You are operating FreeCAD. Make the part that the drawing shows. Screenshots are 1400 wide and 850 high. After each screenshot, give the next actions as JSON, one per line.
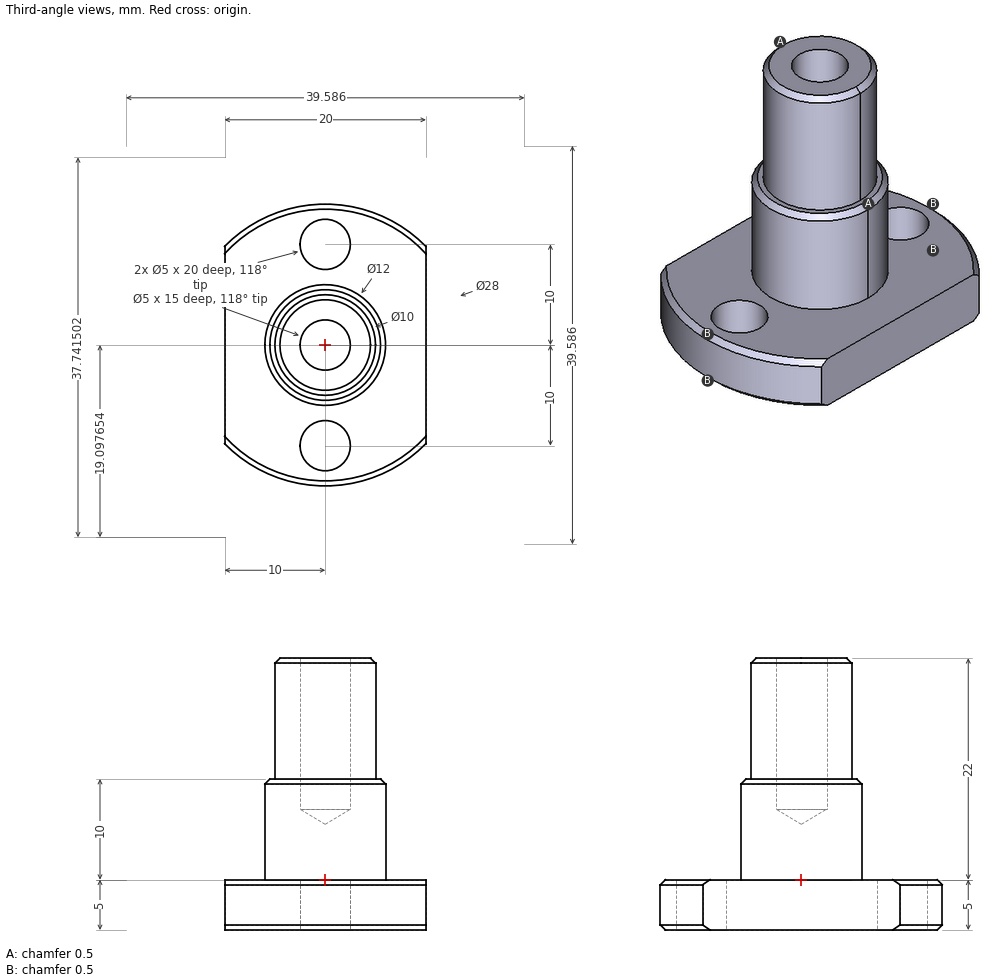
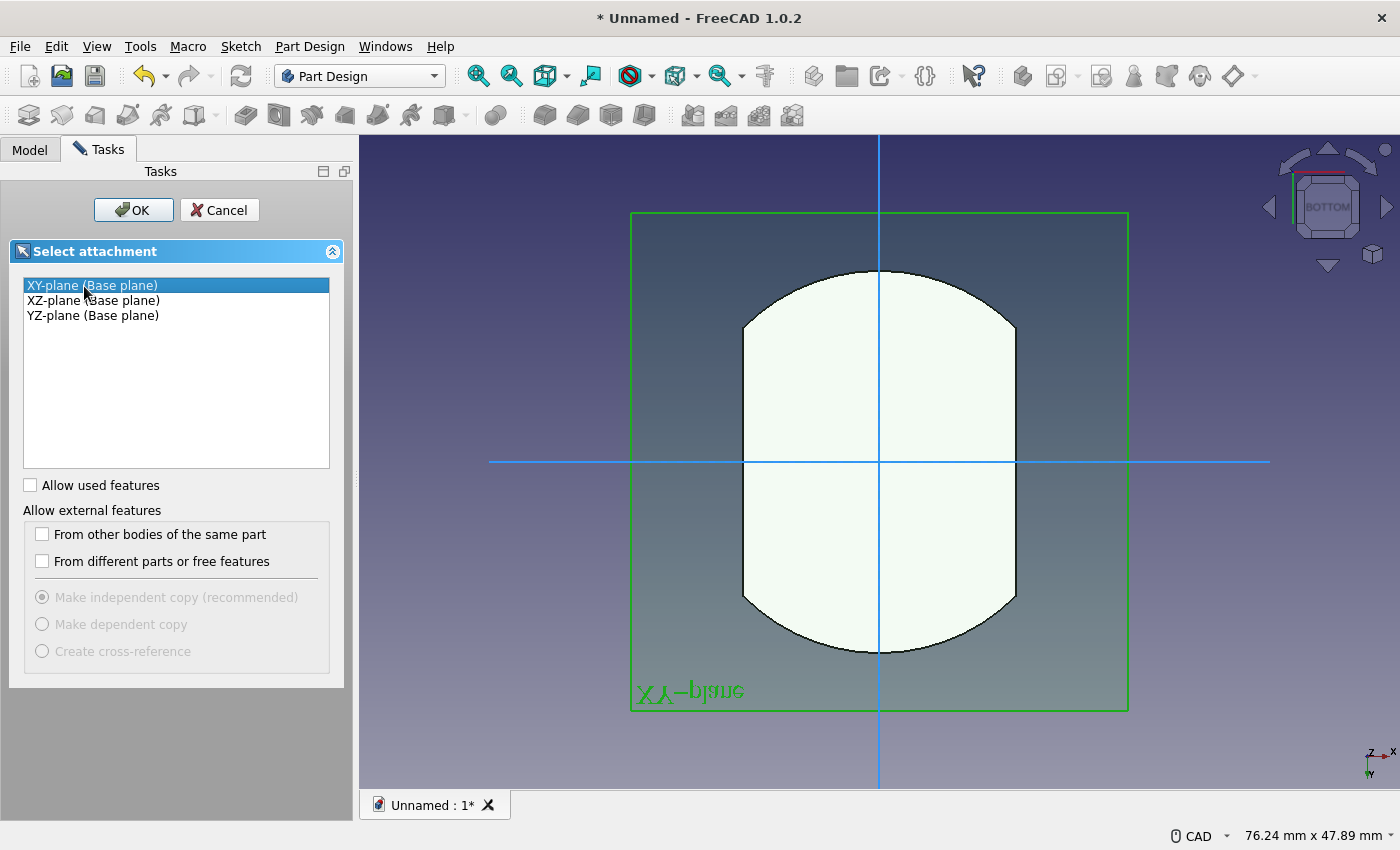
{"action": "left_click", "coordinate": [134, 210]}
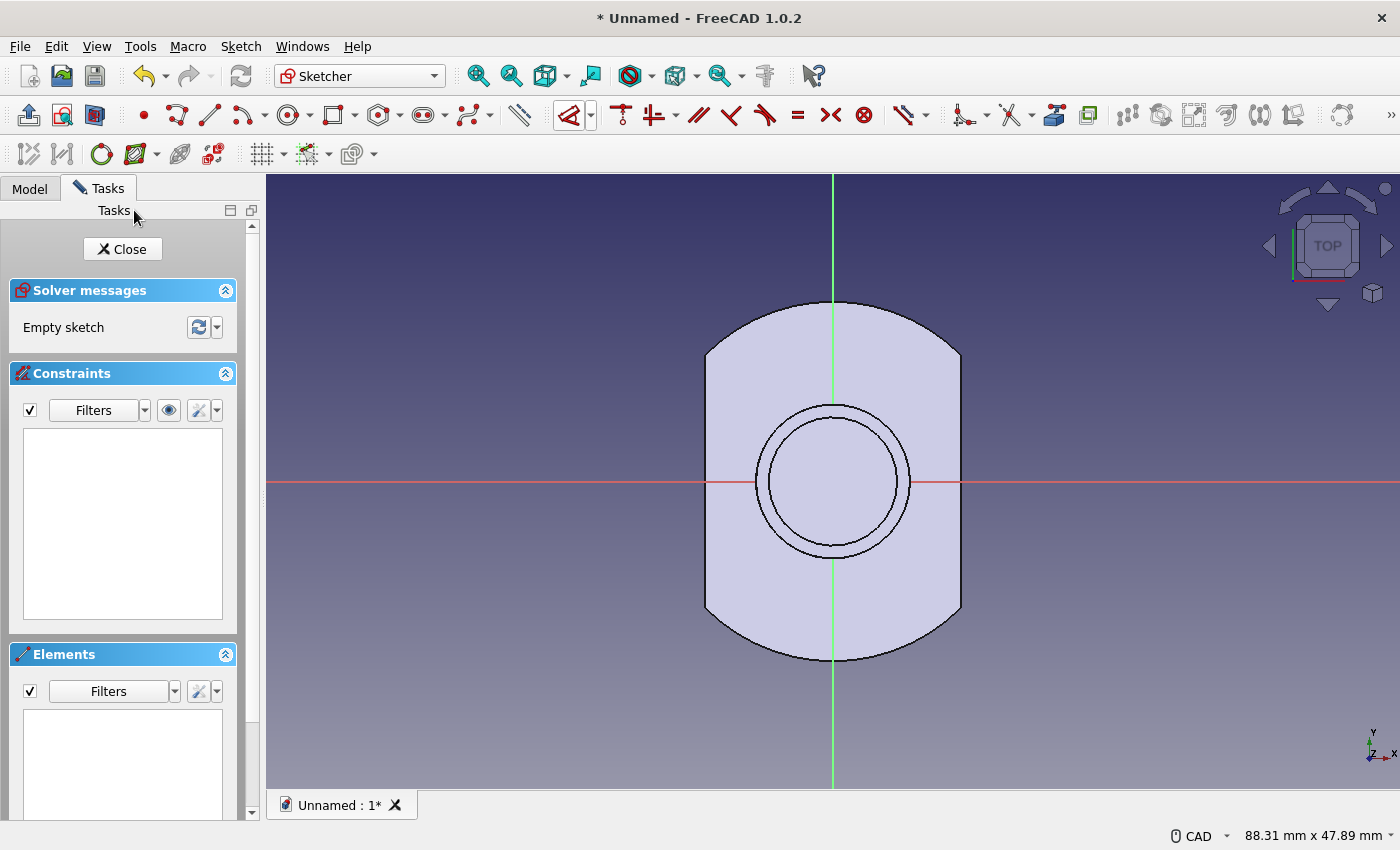
{"action": "key", "text": "q s"}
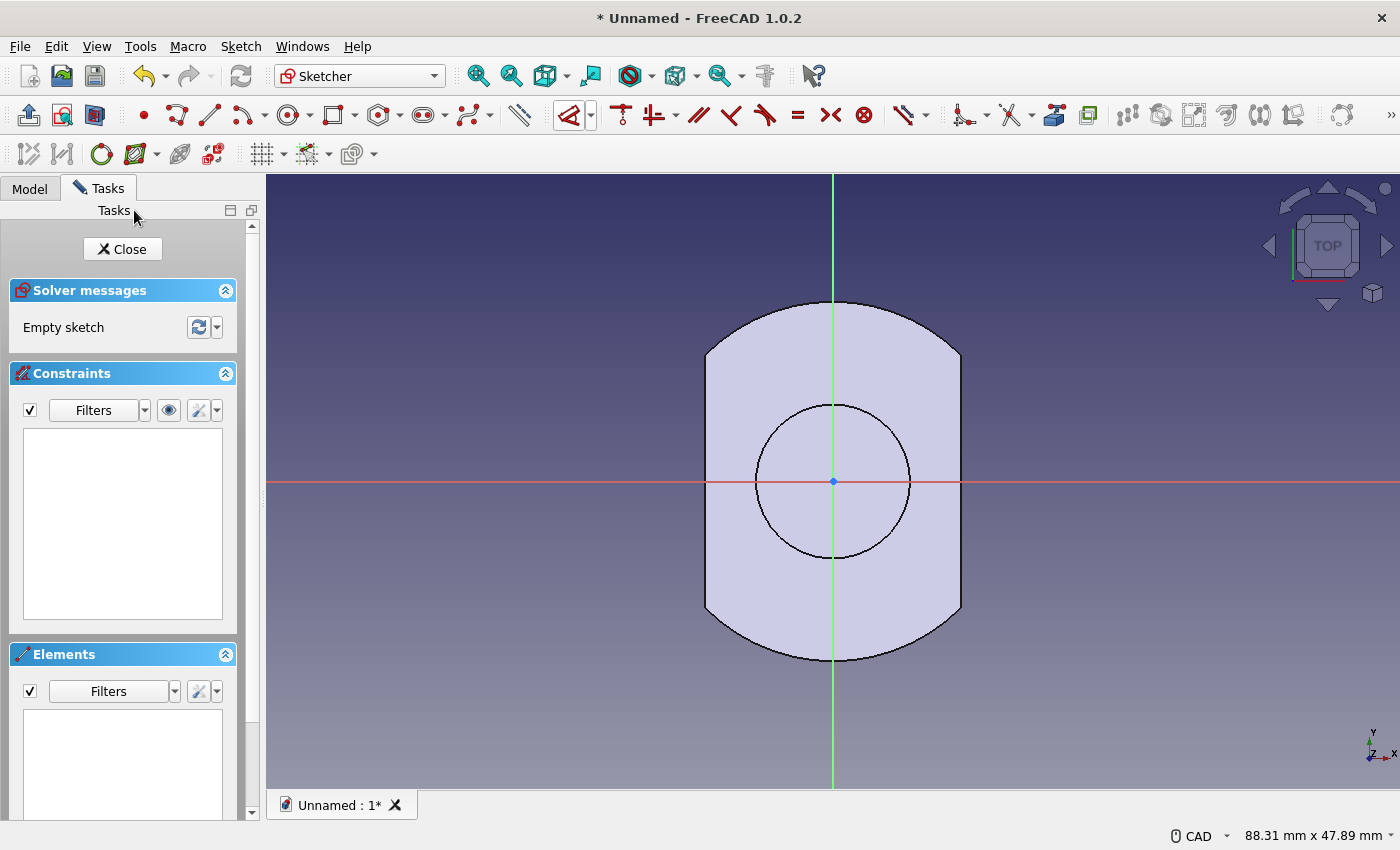
{"action": "left_click", "coordinate": [288, 116]}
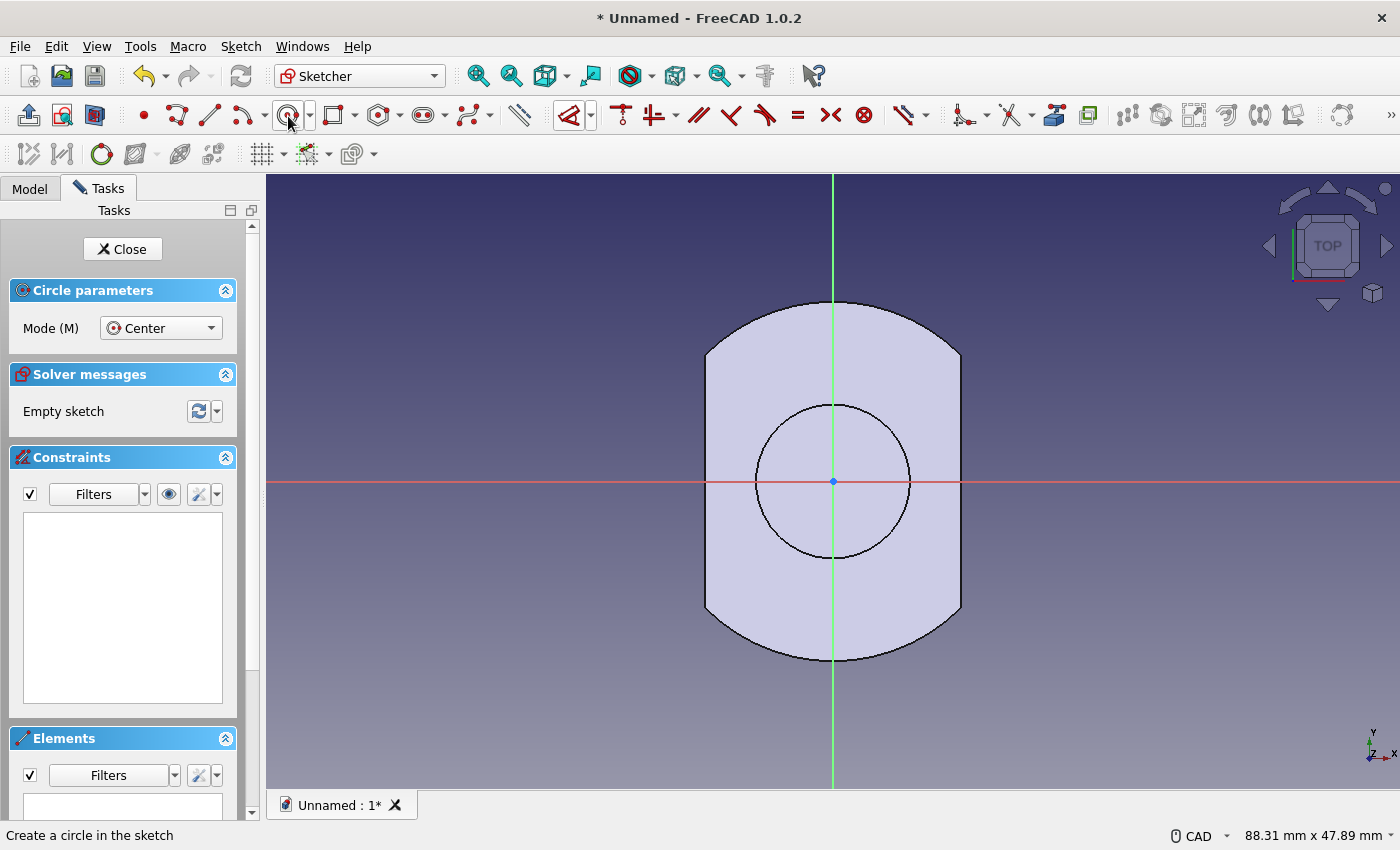
{"action": "left_click", "coordinate": [833, 353]}
{"action": "mouse_move", "coordinate": [856, 330]}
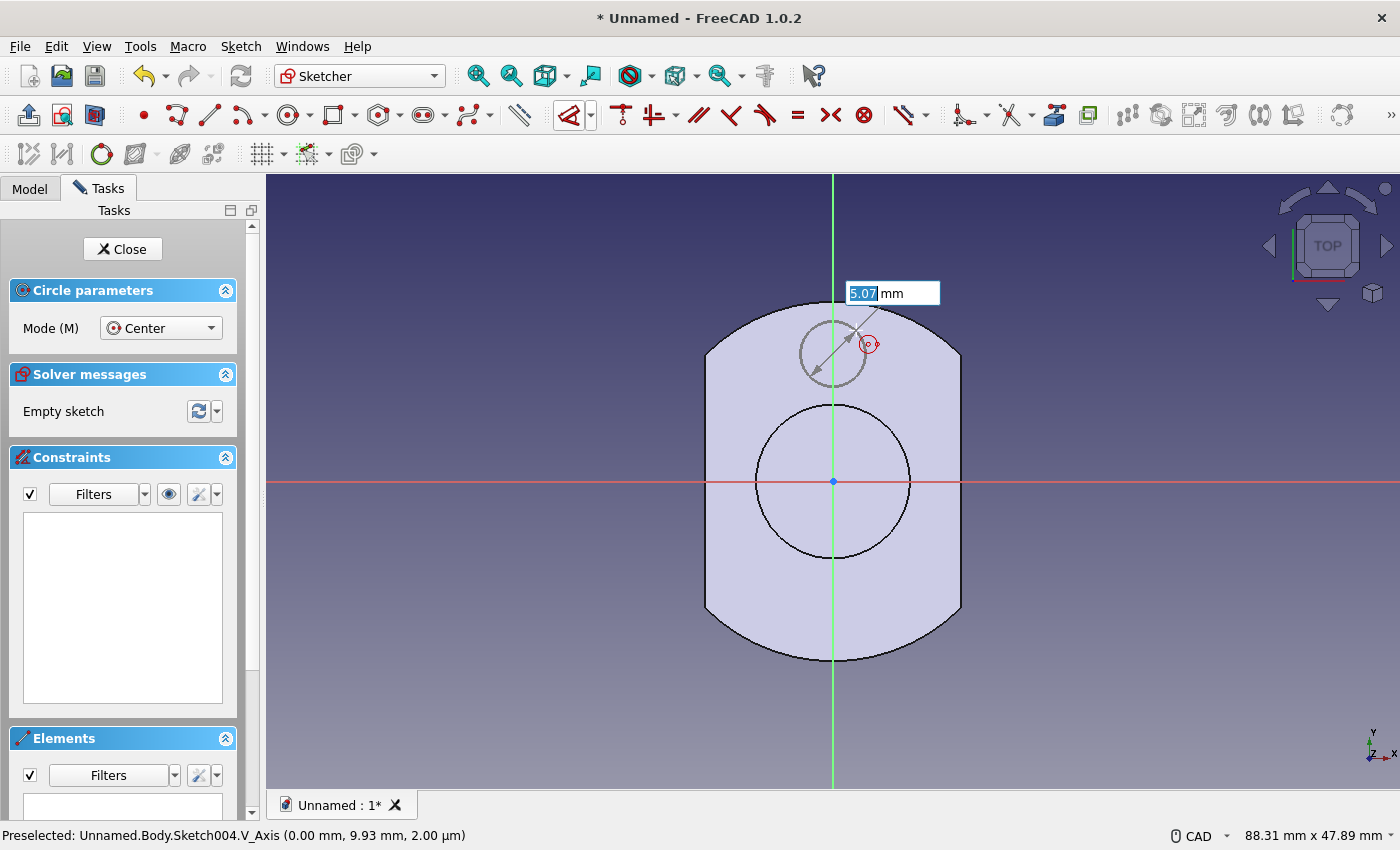
{"action": "type", "text": "5"}
{"action": "key", "text": "Return"}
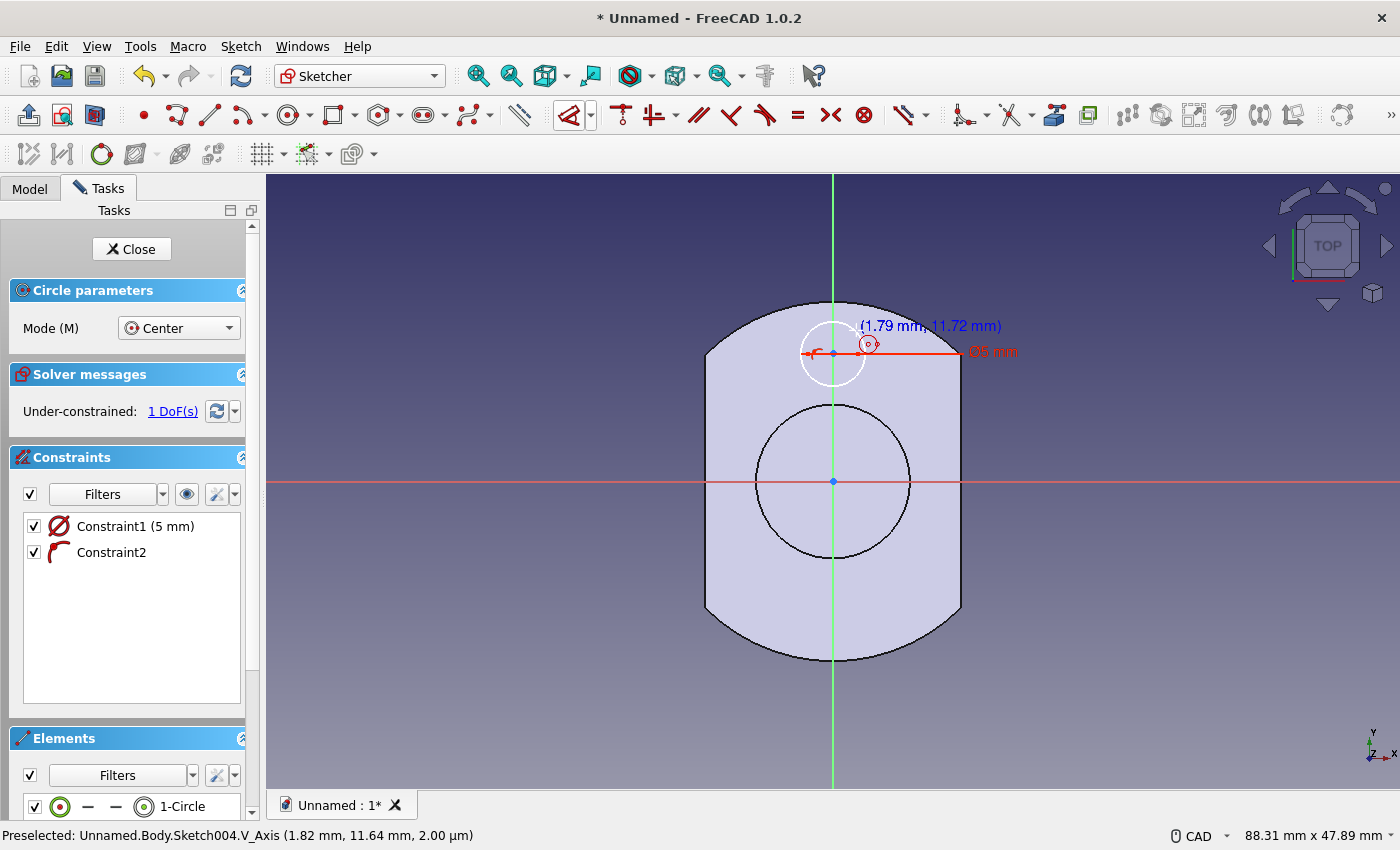
{"action": "left_click", "coordinate": [833, 610]}
{"action": "mouse_move", "coordinate": [856, 587]}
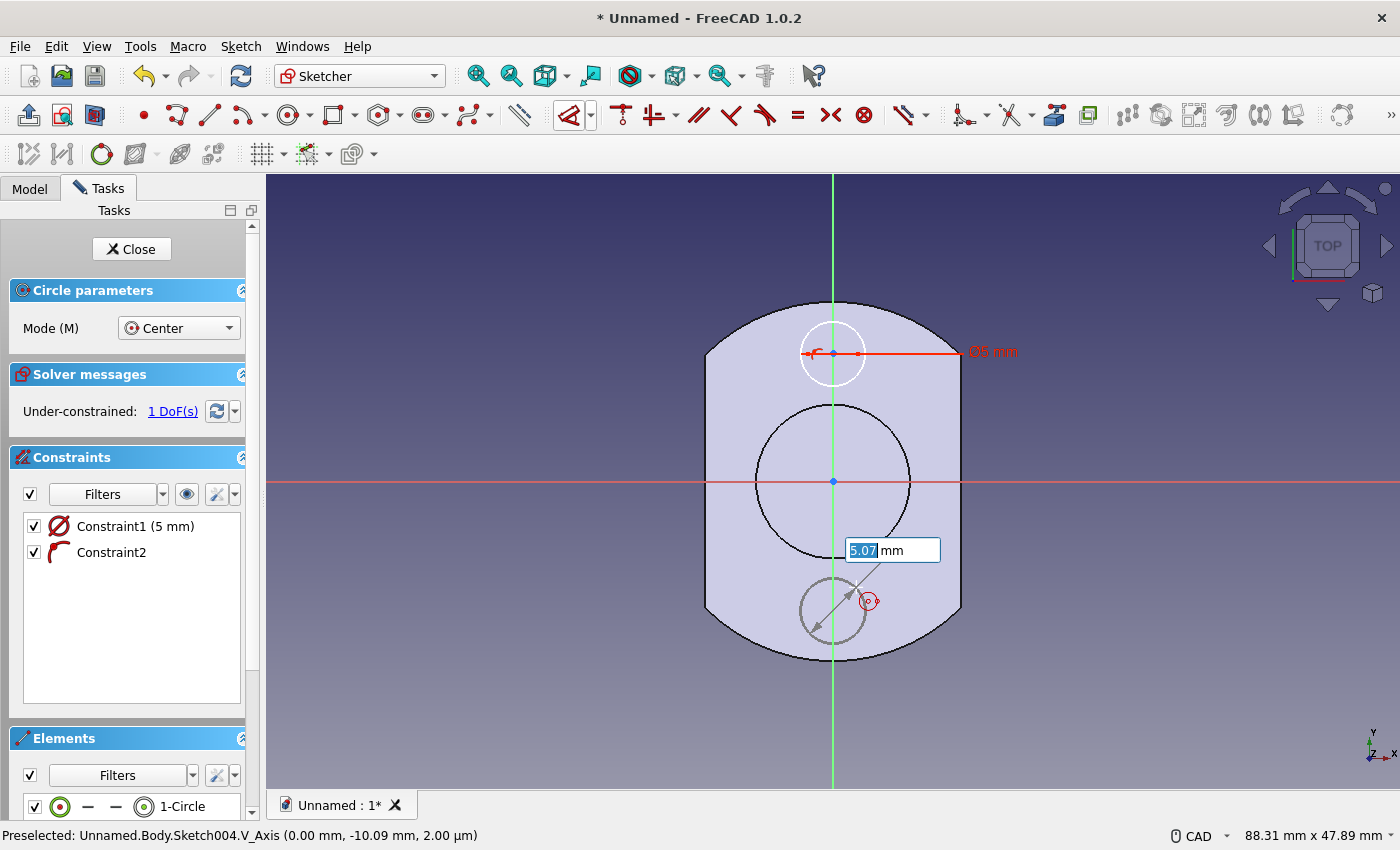
{"action": "type", "text": "5"}
{"action": "key", "text": "Return"}
{"action": "key", "text": "Escape"}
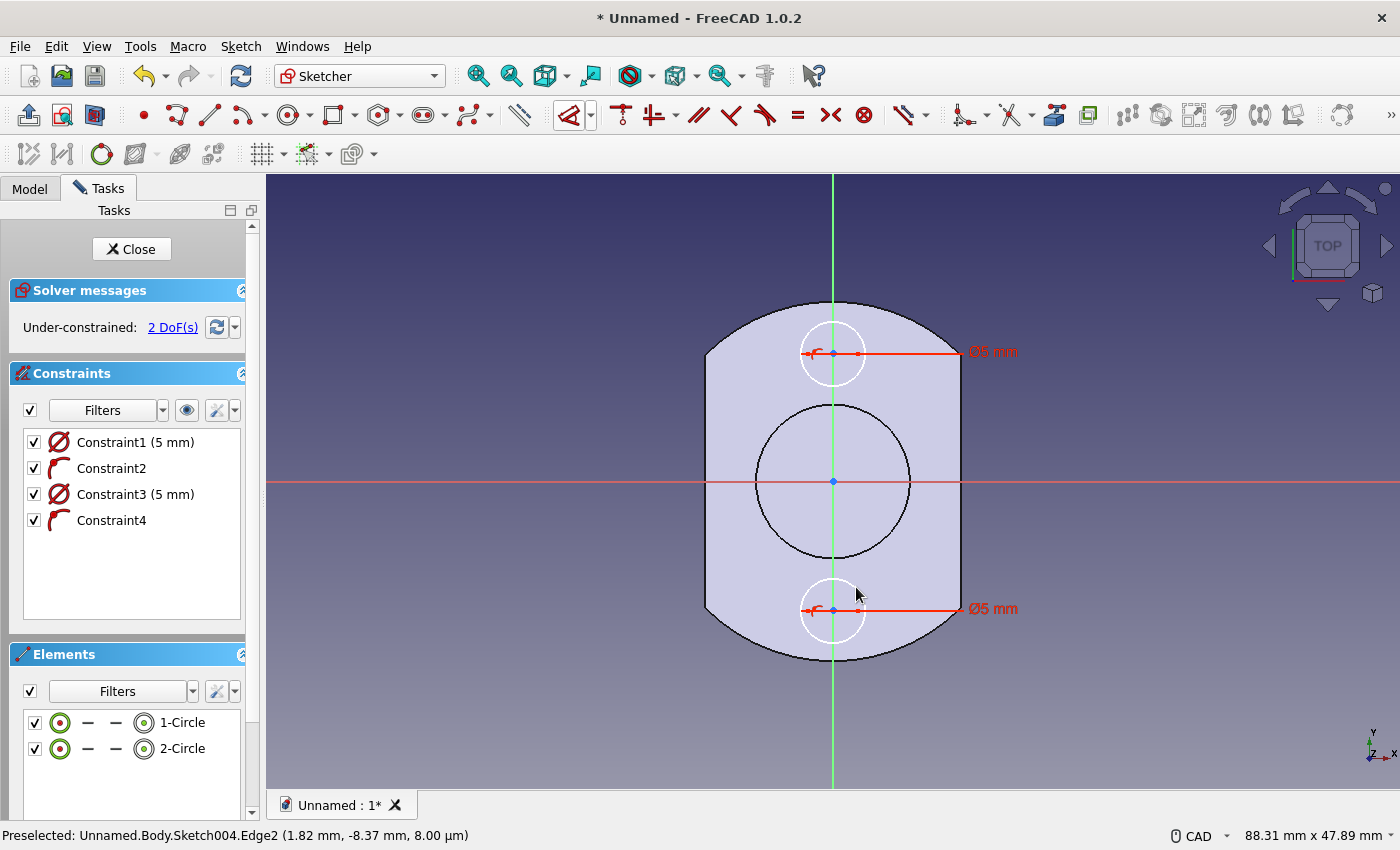
{"action": "left_click", "coordinate": [833, 354]}